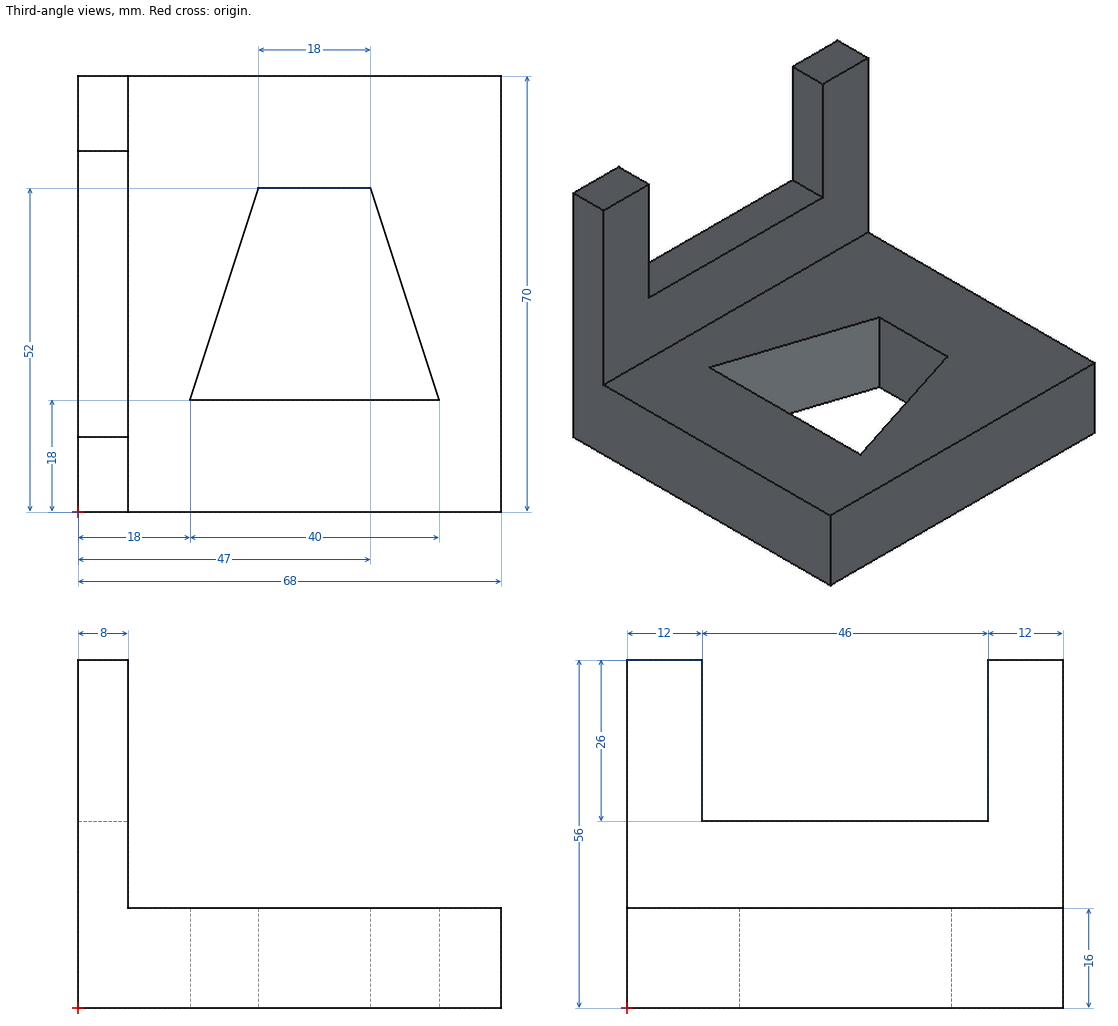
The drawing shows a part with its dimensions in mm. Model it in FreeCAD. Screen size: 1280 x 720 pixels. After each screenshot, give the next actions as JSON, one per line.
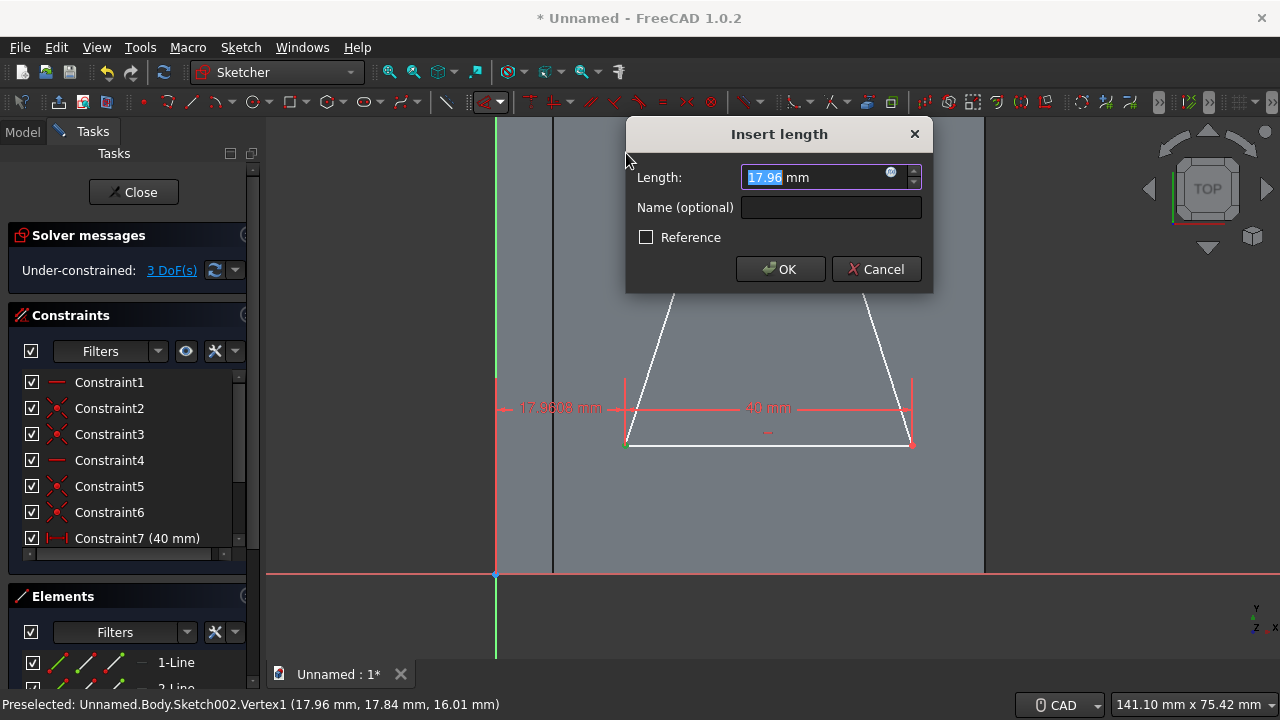
{"action": "type", "text": "18"}
{"action": "key", "text": "Return"}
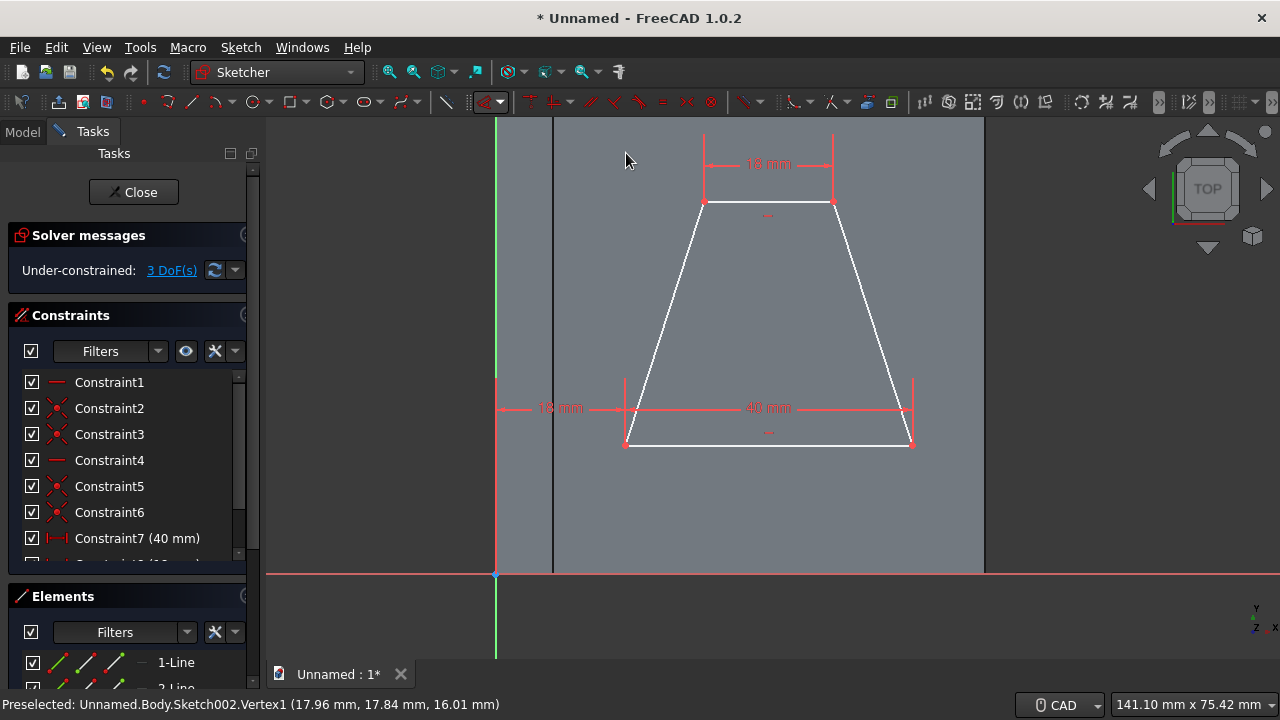
{"action": "left_click", "coordinate": [625, 446]}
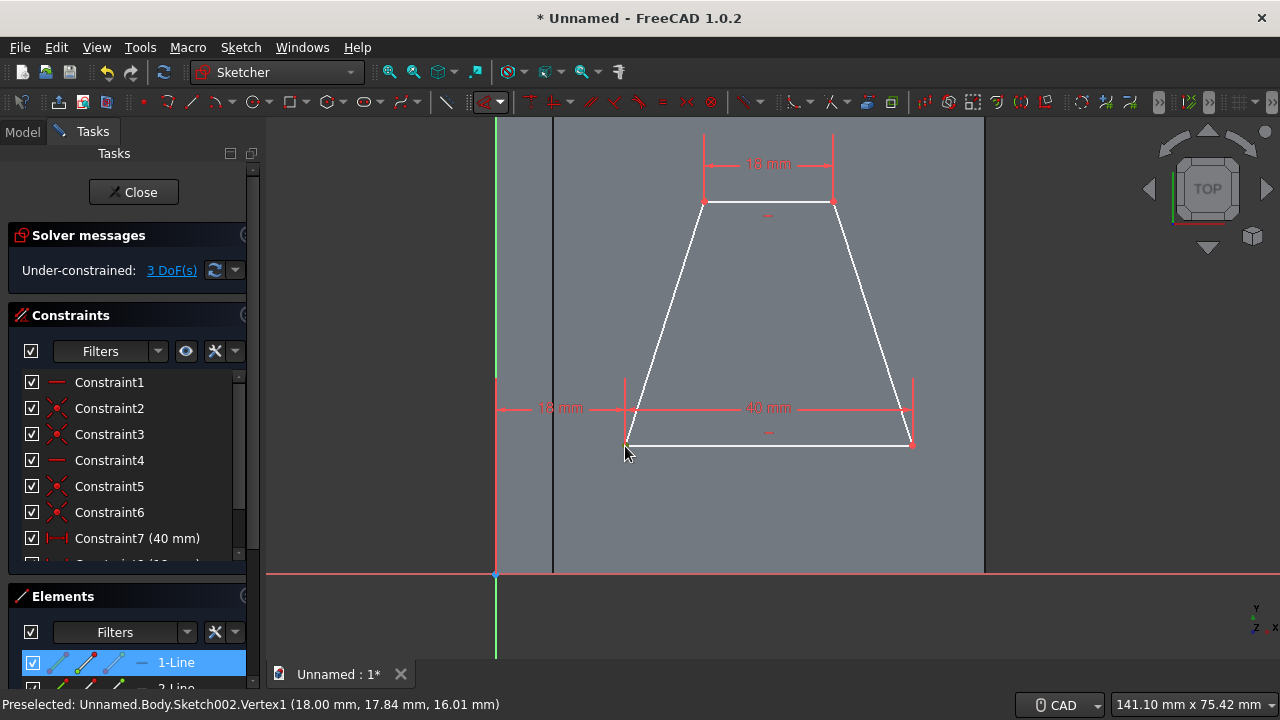
{"action": "key", "text": "i"}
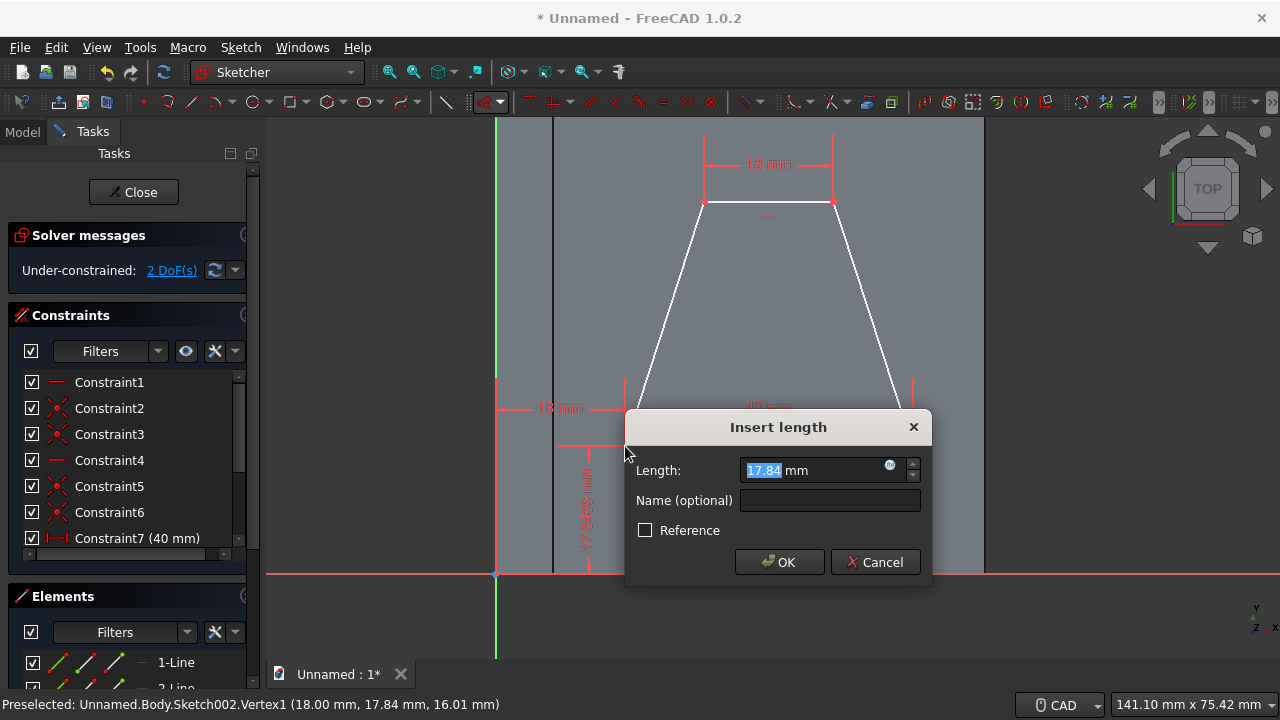
{"action": "type", "text": "18"}
{"action": "key", "text": "Return"}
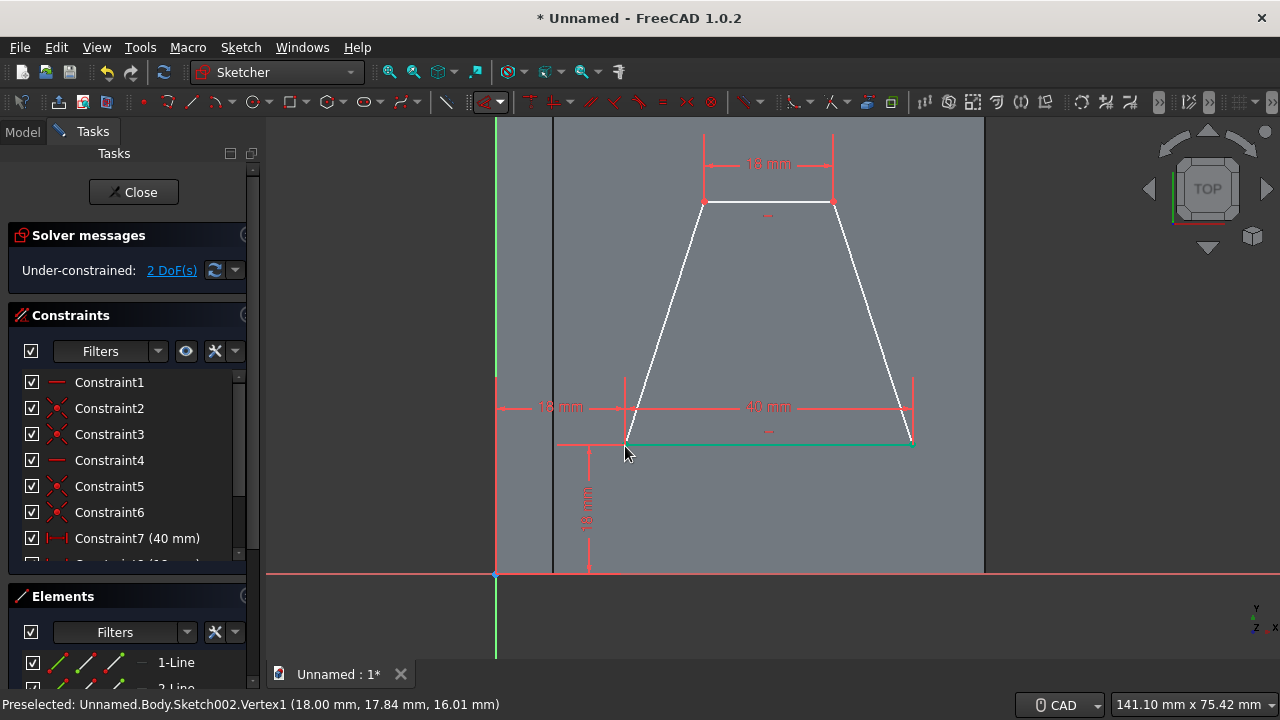
{"action": "left_click", "coordinate": [833, 202]}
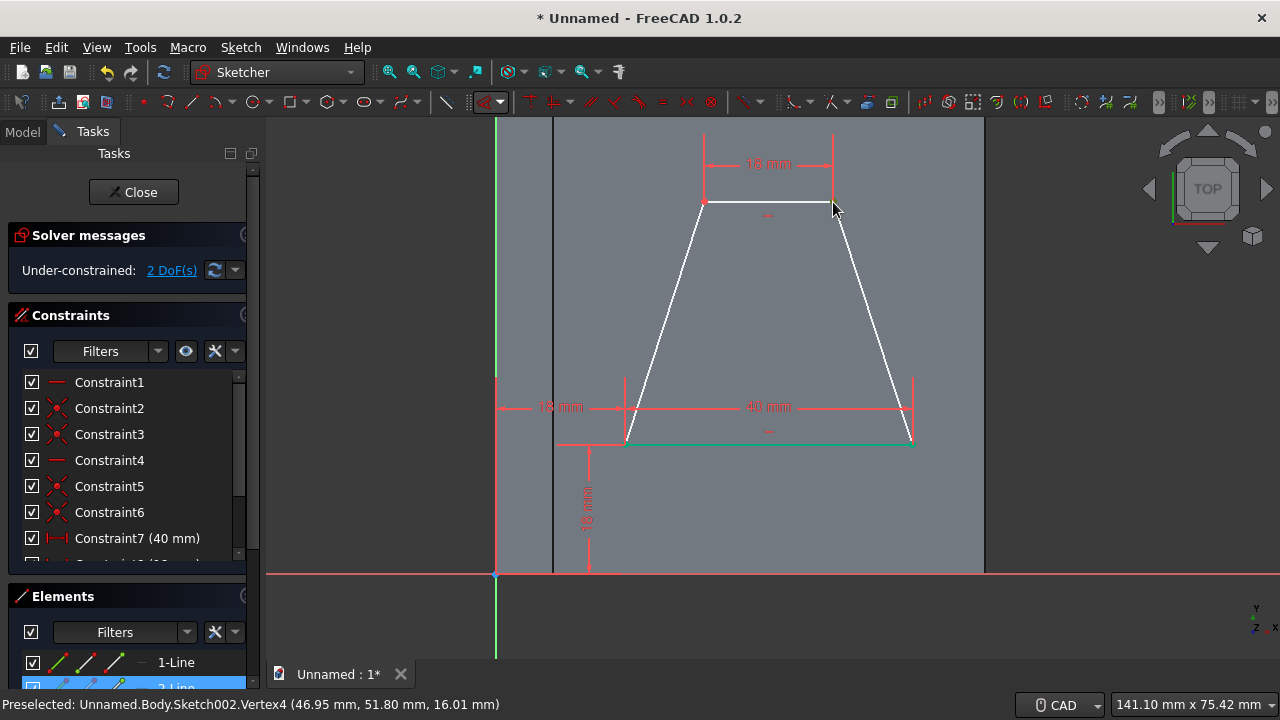
{"action": "key", "text": "l"}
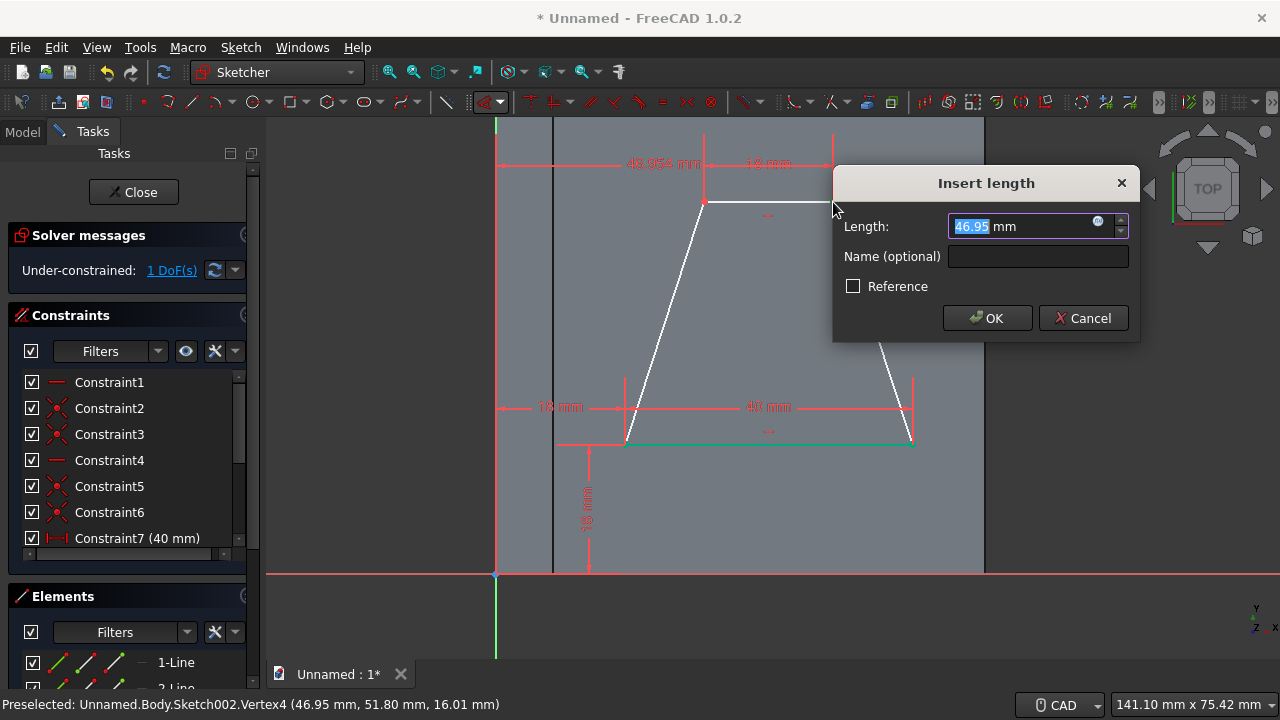
{"action": "type", "text": "47"}
{"action": "key", "text": "Return"}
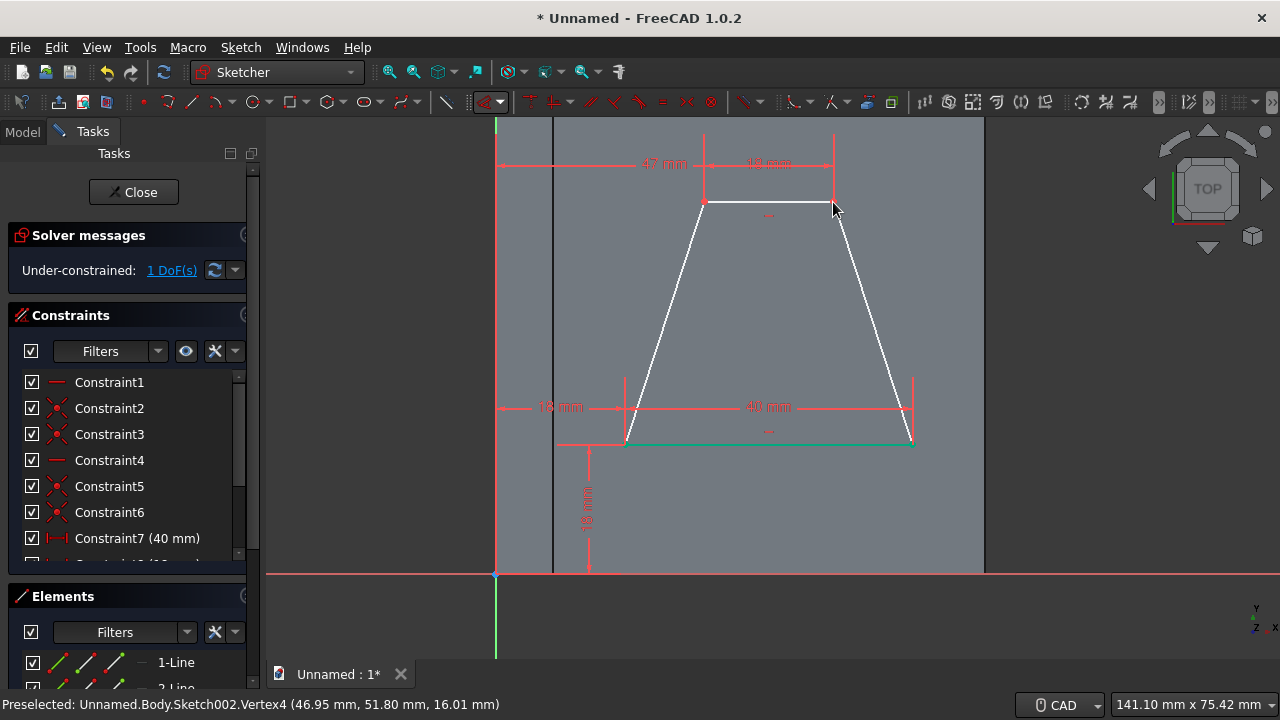
{"action": "left_click", "coordinate": [834, 202]}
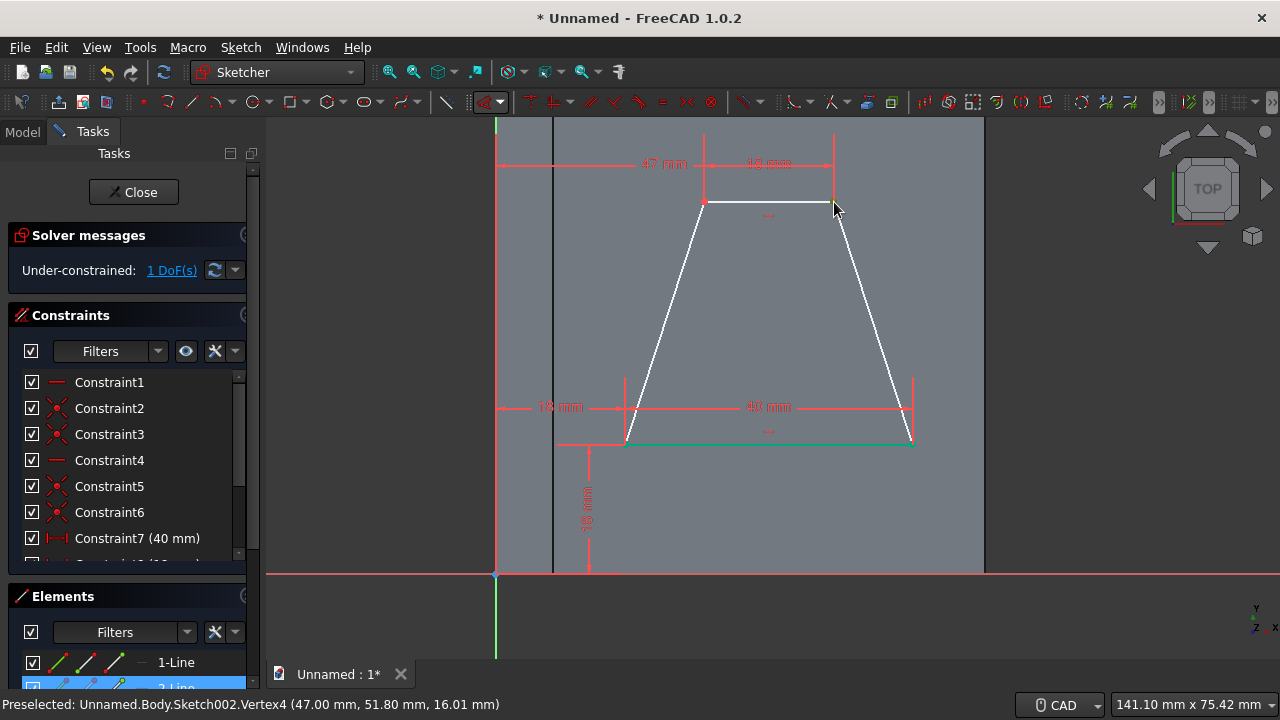
{"action": "left_click", "coordinate": [502, 102]}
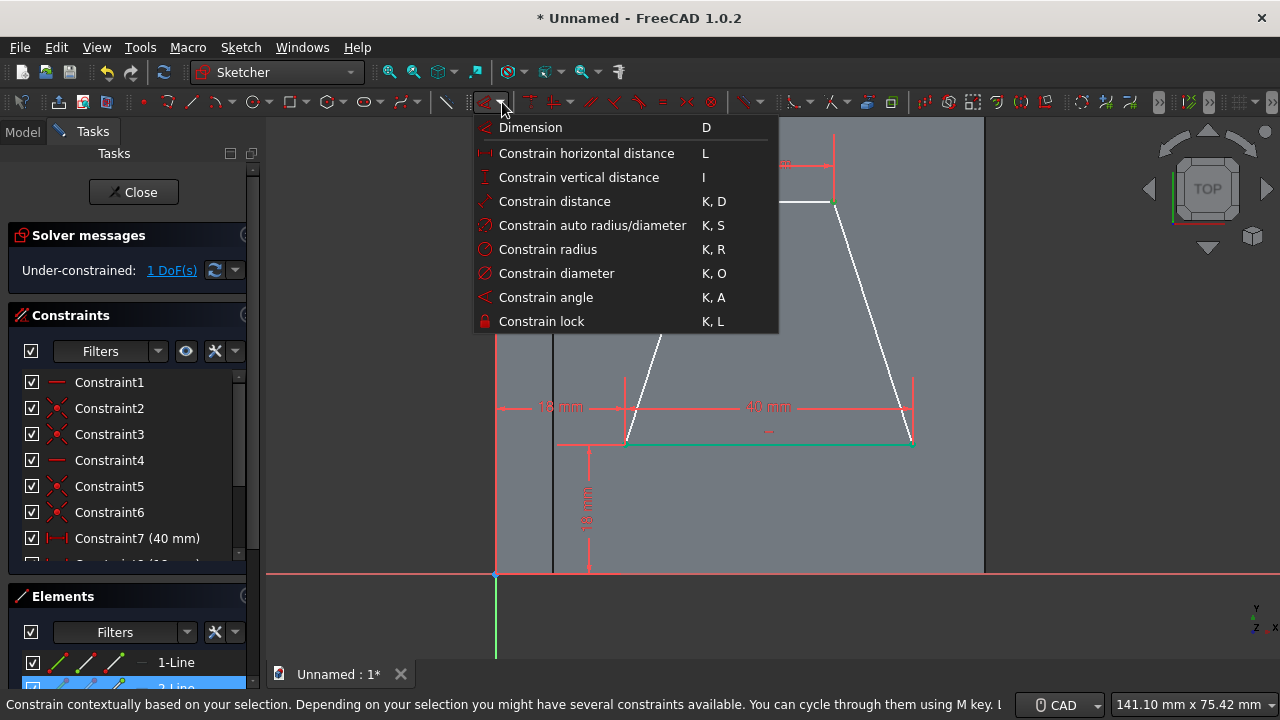
{"action": "left_click", "coordinate": [626, 177]}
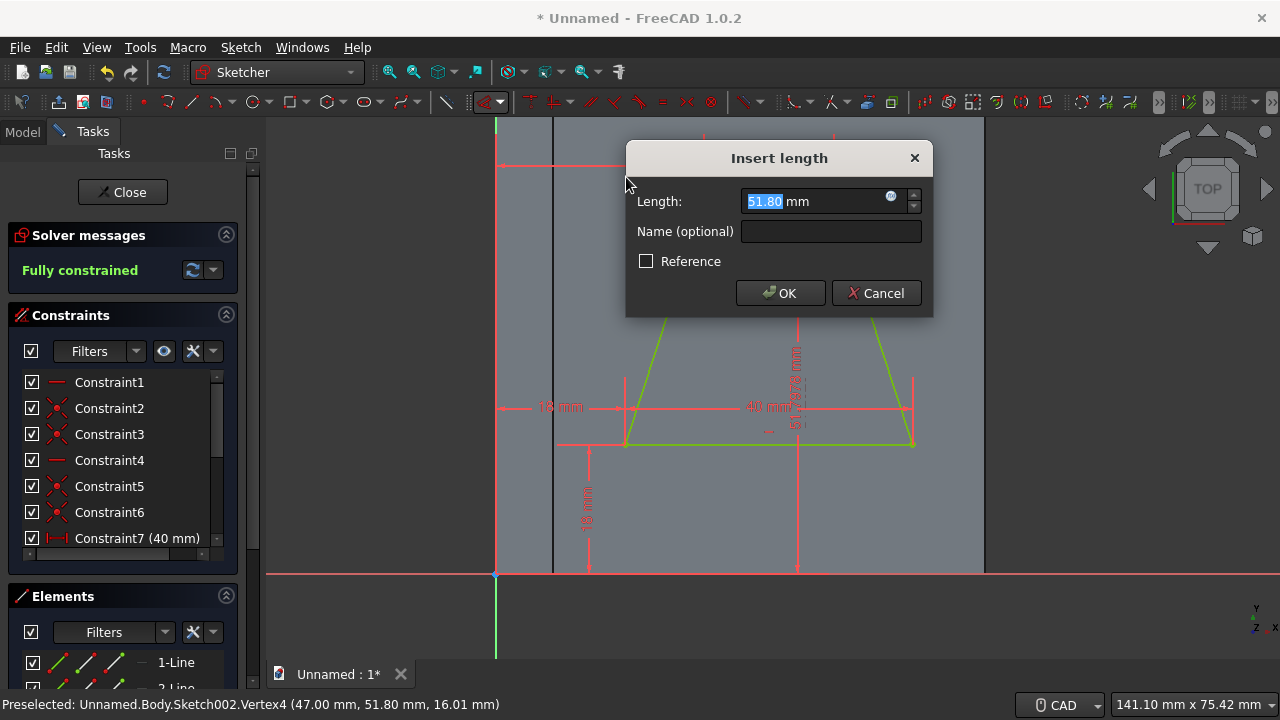
{"action": "type", "text": "52"}
{"action": "key", "text": "Return"}